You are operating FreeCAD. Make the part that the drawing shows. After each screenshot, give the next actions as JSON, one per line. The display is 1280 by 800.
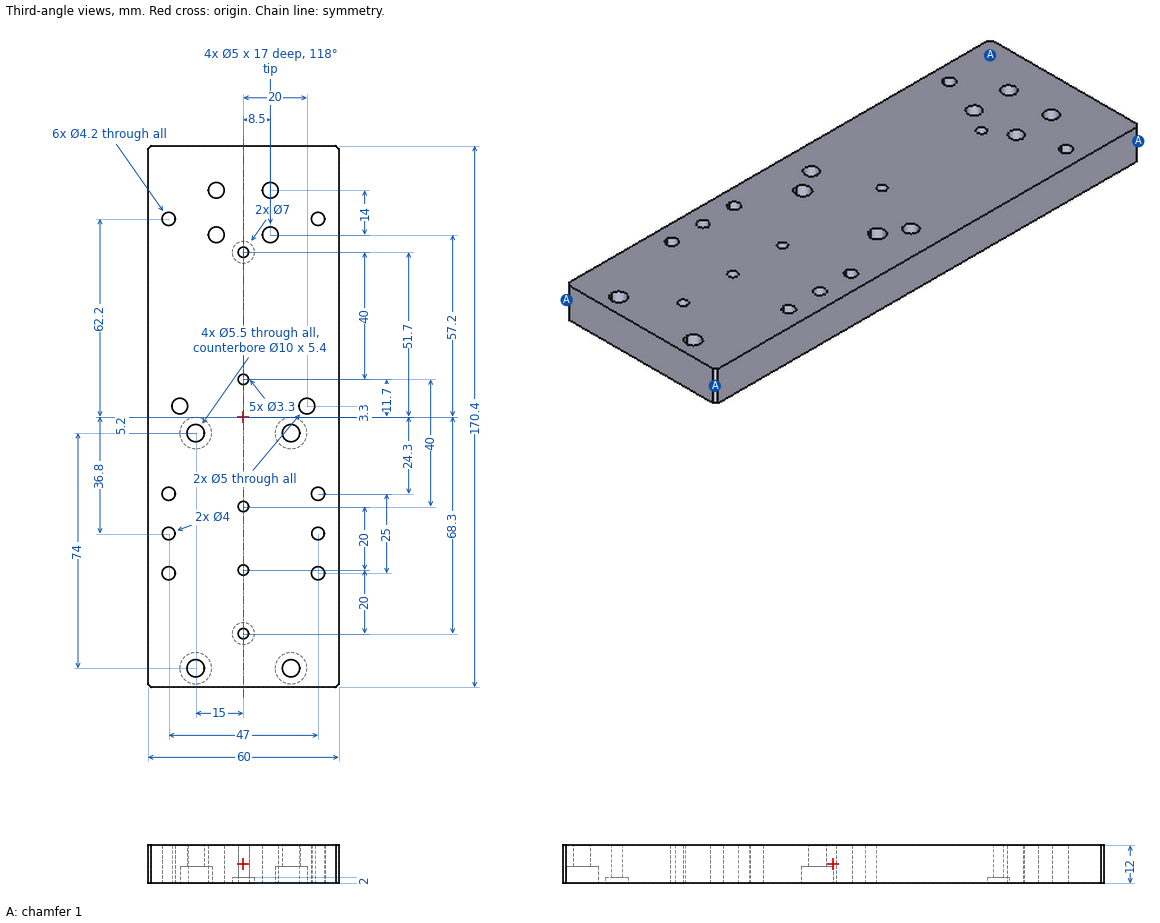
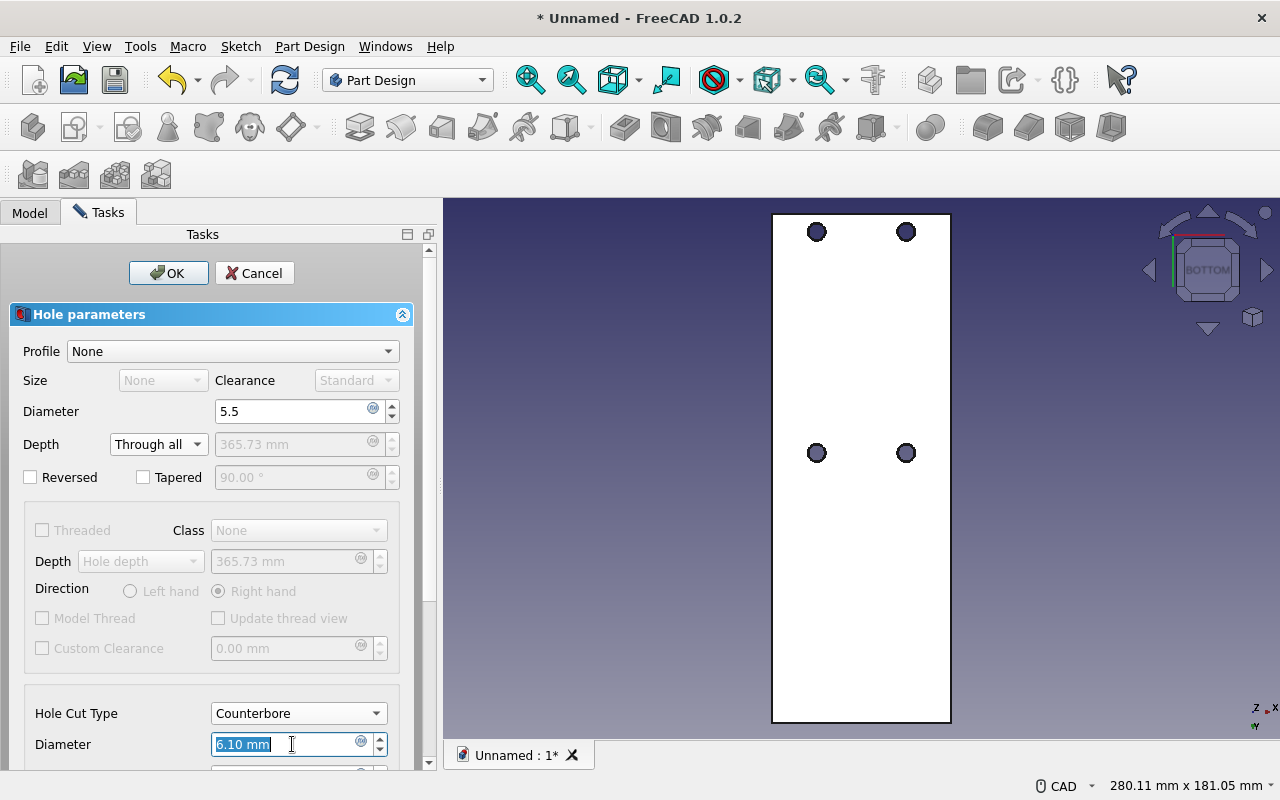
{"action": "type", "text": "10"}
{"action": "key", "text": "Tab"}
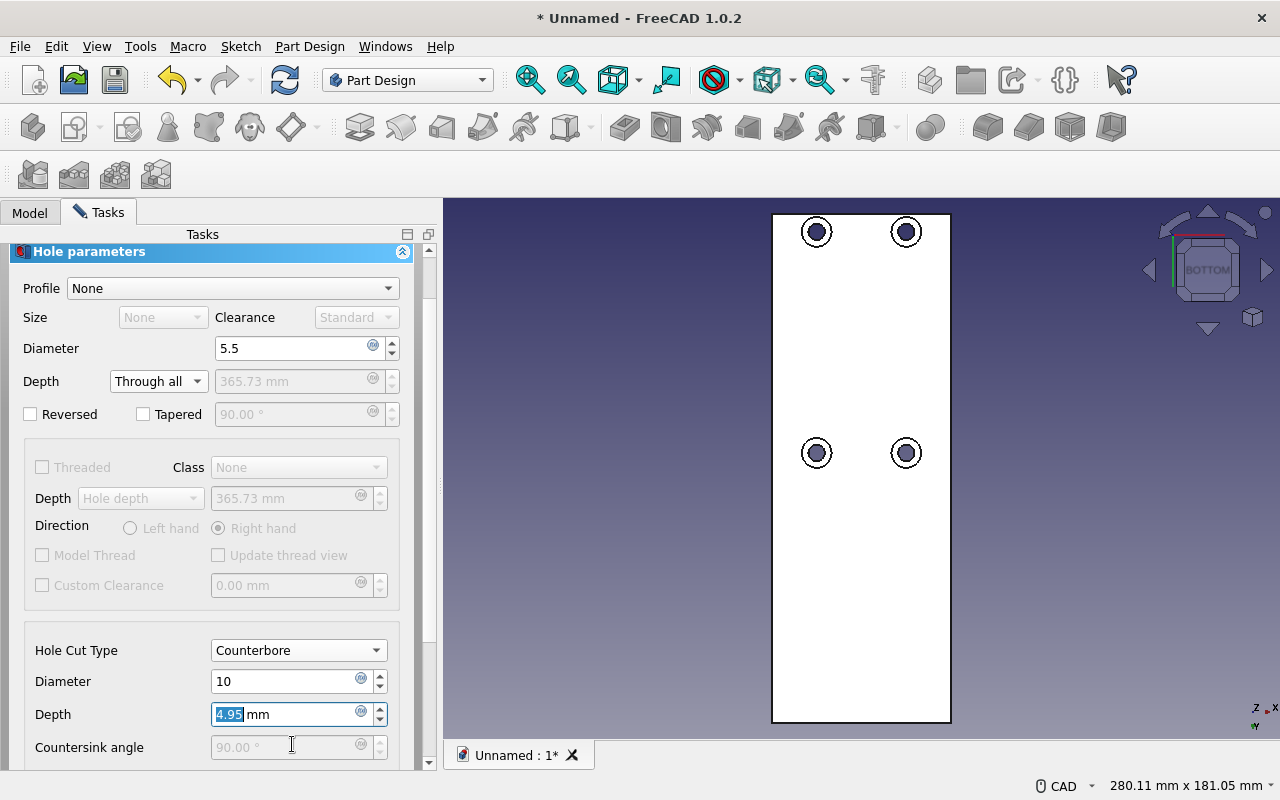
{"action": "type", "text": "5.4"}
{"action": "key", "text": "Tab"}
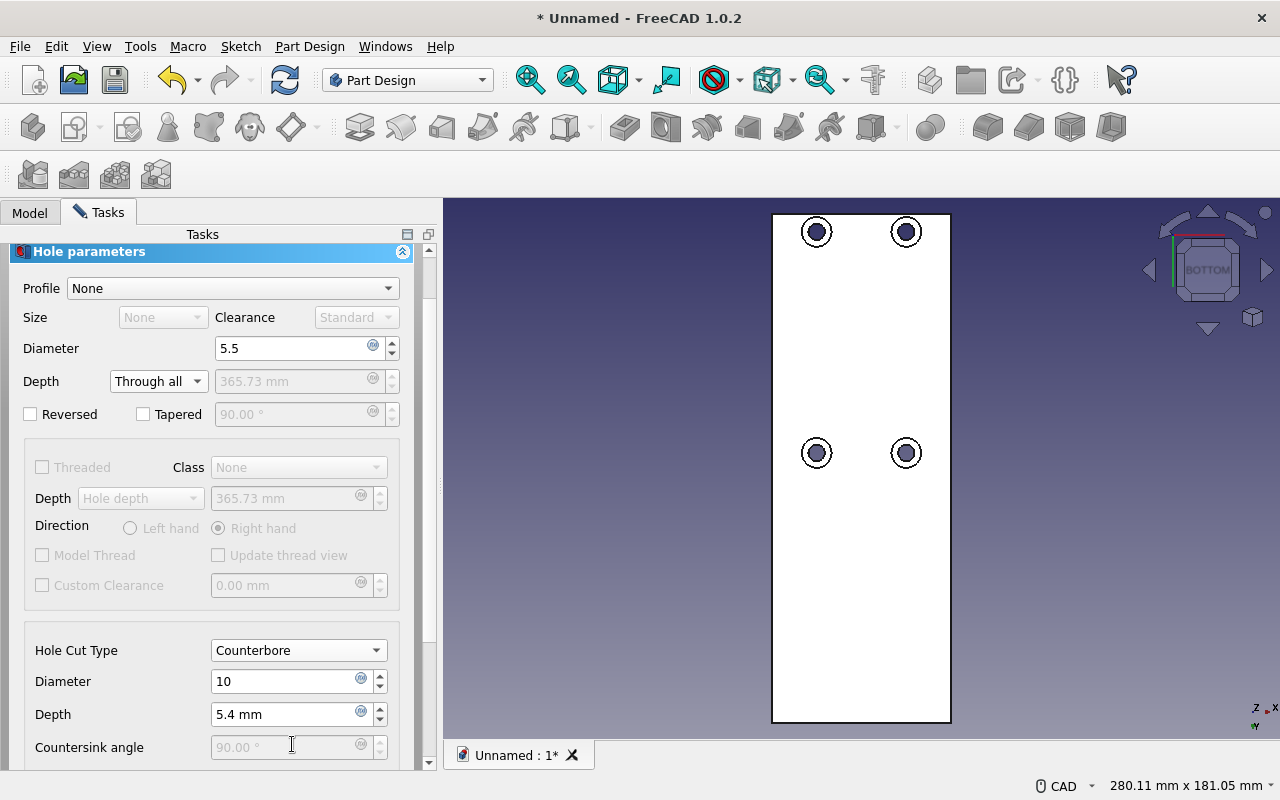
{"action": "scroll", "coordinate": [429, 507], "scroll_direction": "up", "scroll_amount": 2}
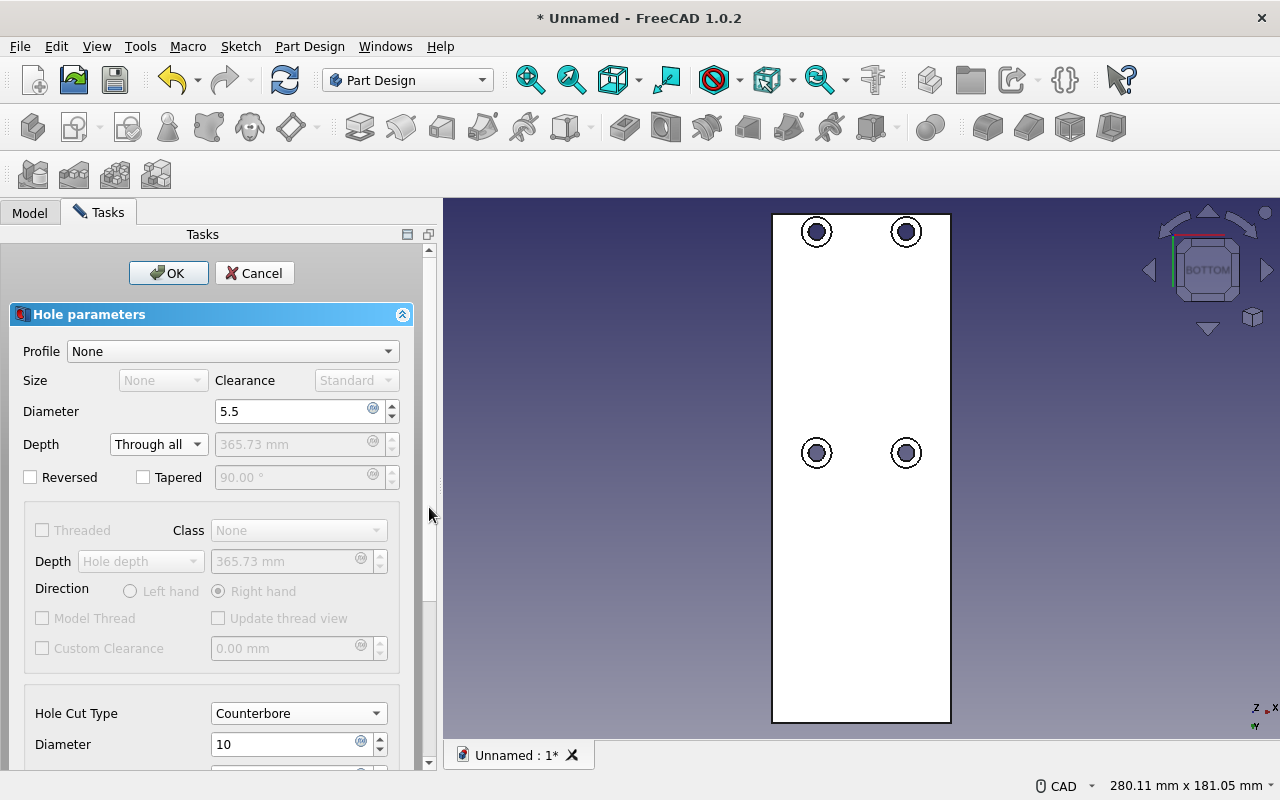
{"action": "left_click", "coordinate": [169, 273]}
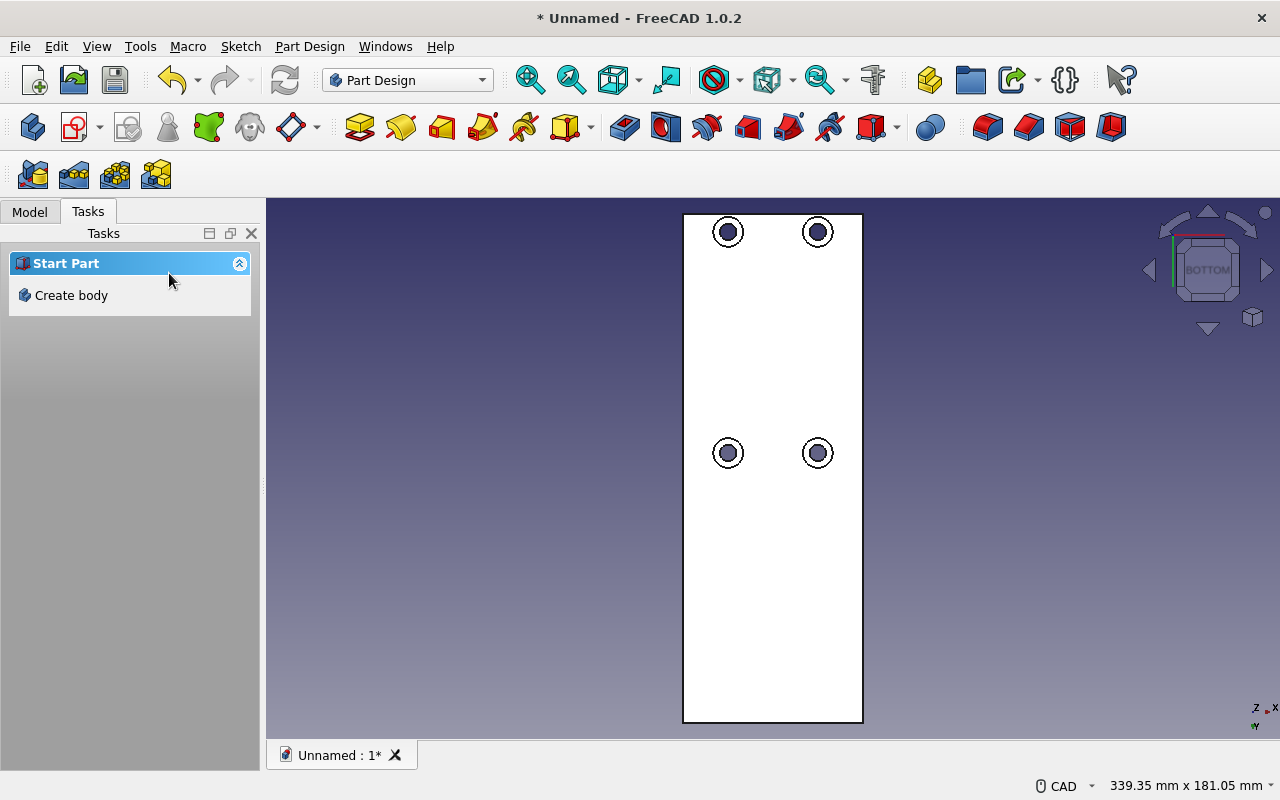
{"action": "key", "text": "0"}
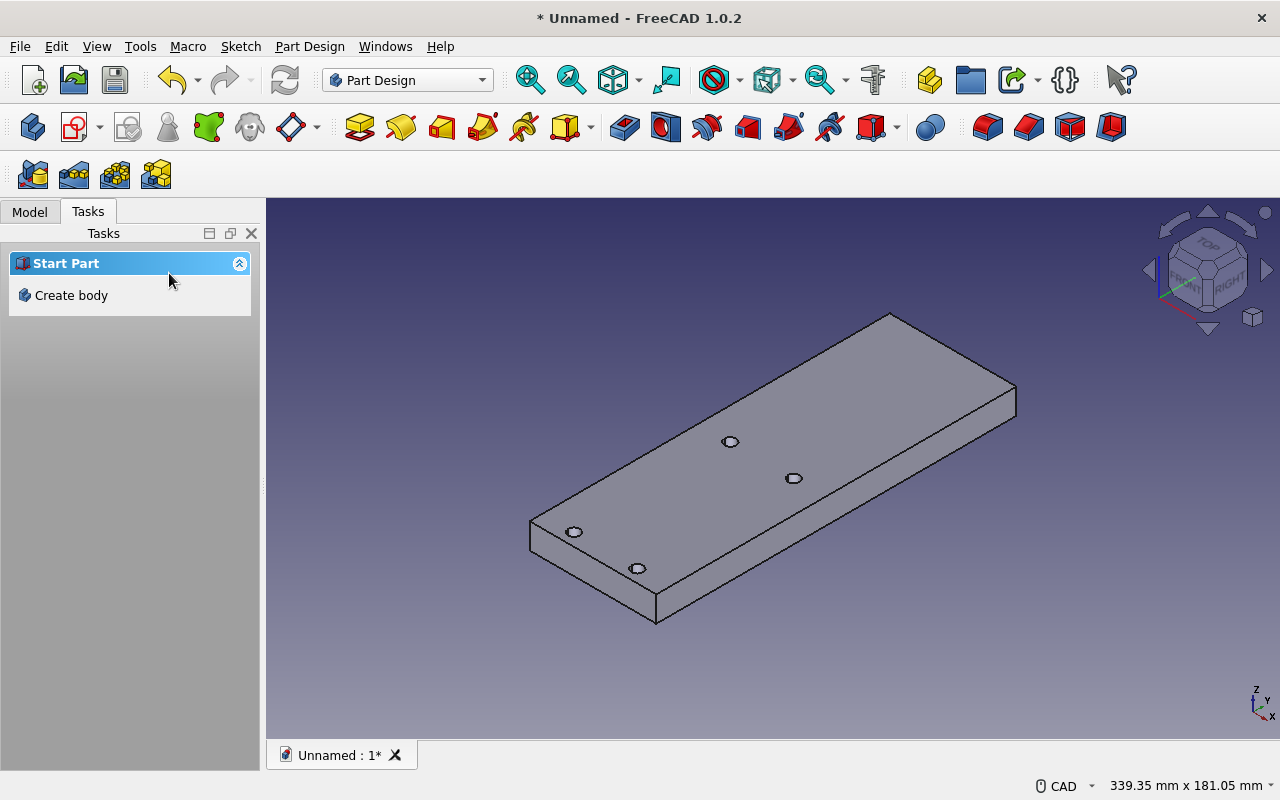
{"action": "left_click", "coordinate": [876, 393]}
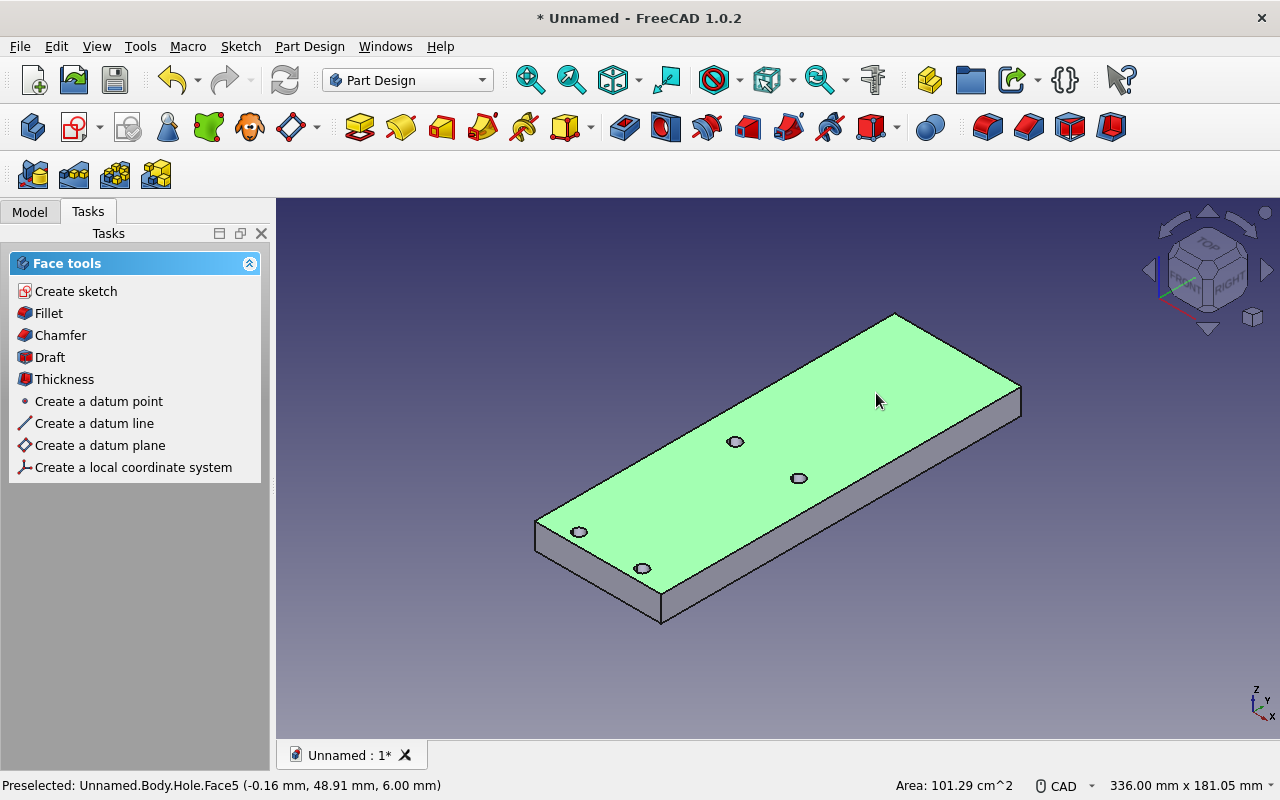
{"action": "left_click", "coordinate": [74, 128]}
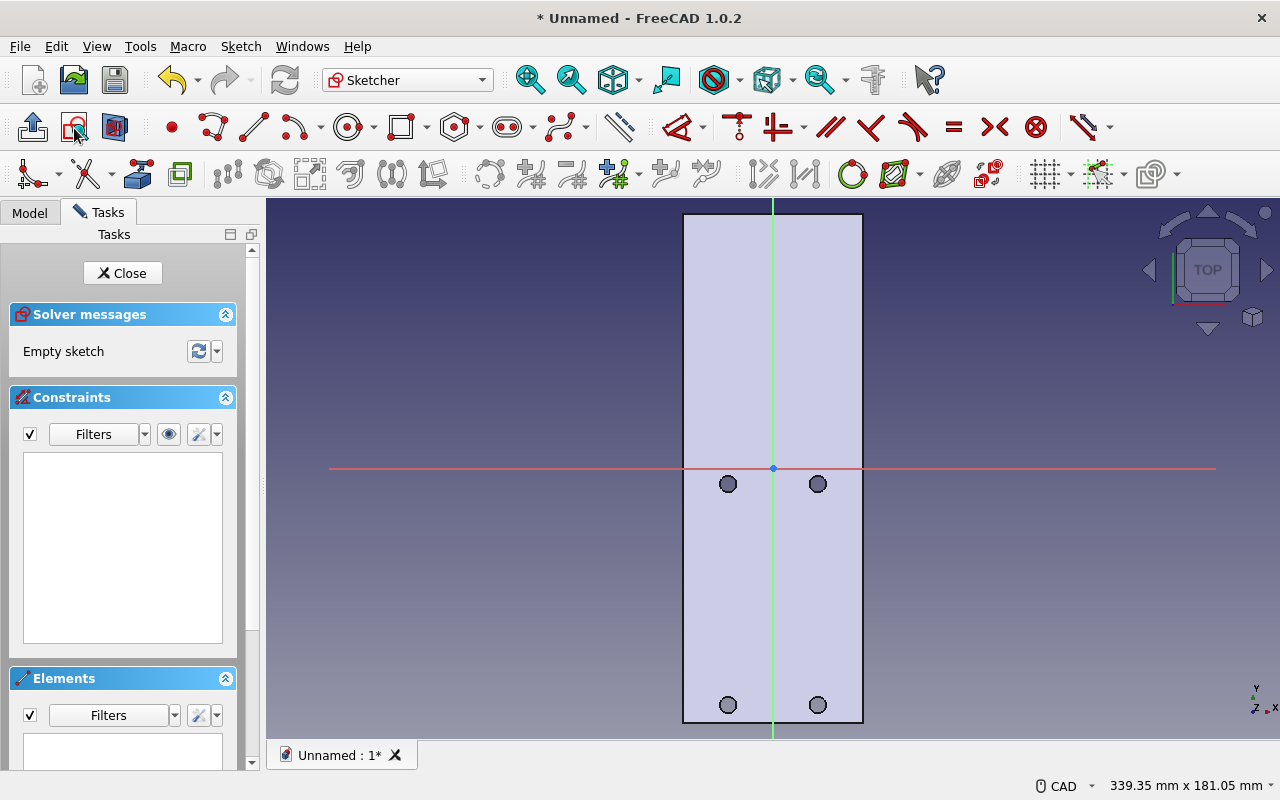
{"action": "scroll", "coordinate": [795, 457], "scroll_direction": "up", "scroll_amount": 7}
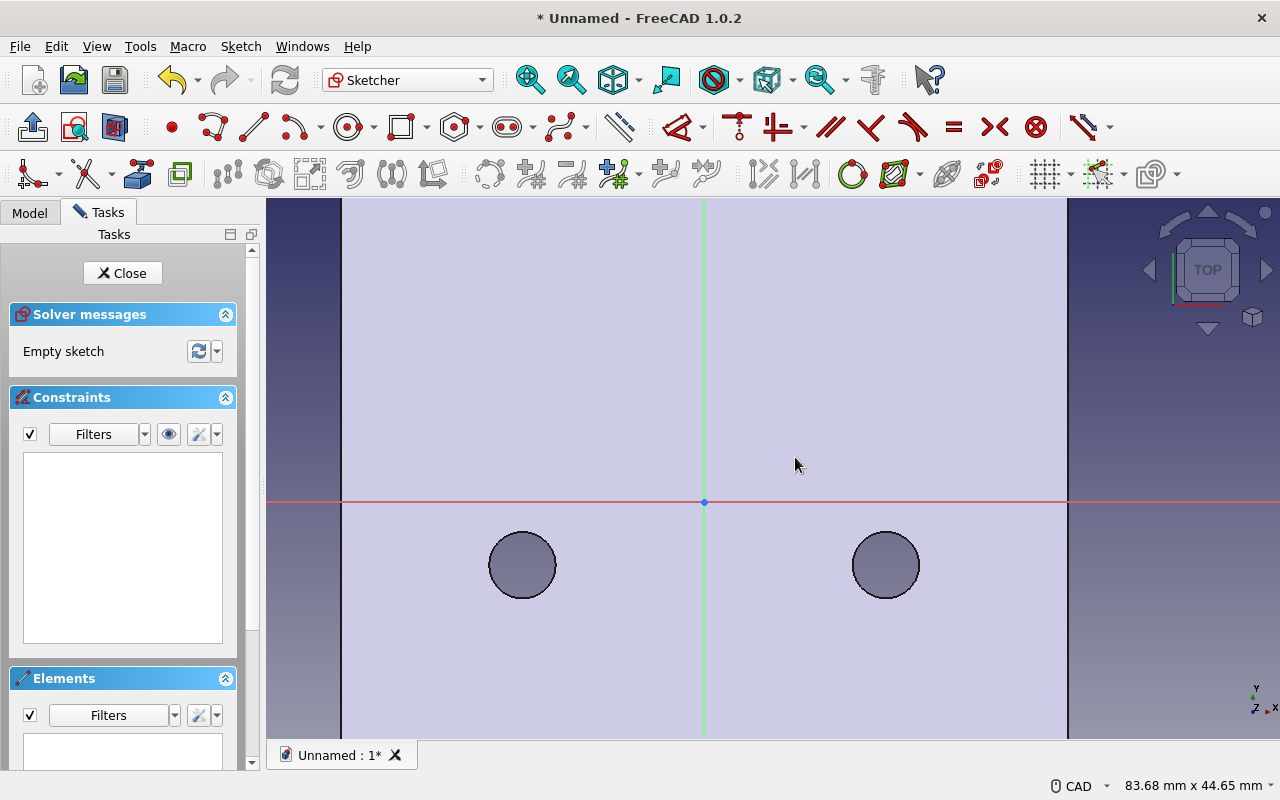
{"action": "left_click", "coordinate": [348, 128]}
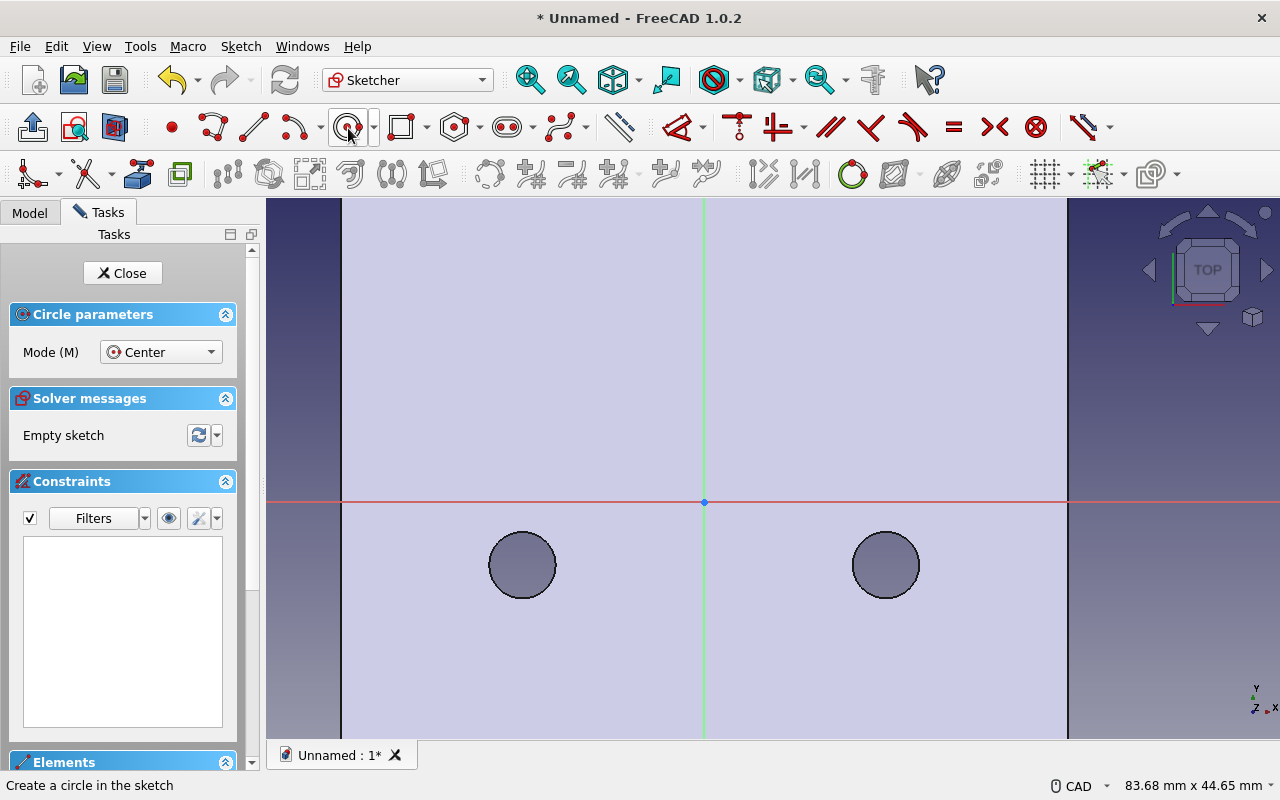
{"action": "left_click", "coordinate": [947, 462]}
{"action": "left_click", "coordinate": [968, 441]}